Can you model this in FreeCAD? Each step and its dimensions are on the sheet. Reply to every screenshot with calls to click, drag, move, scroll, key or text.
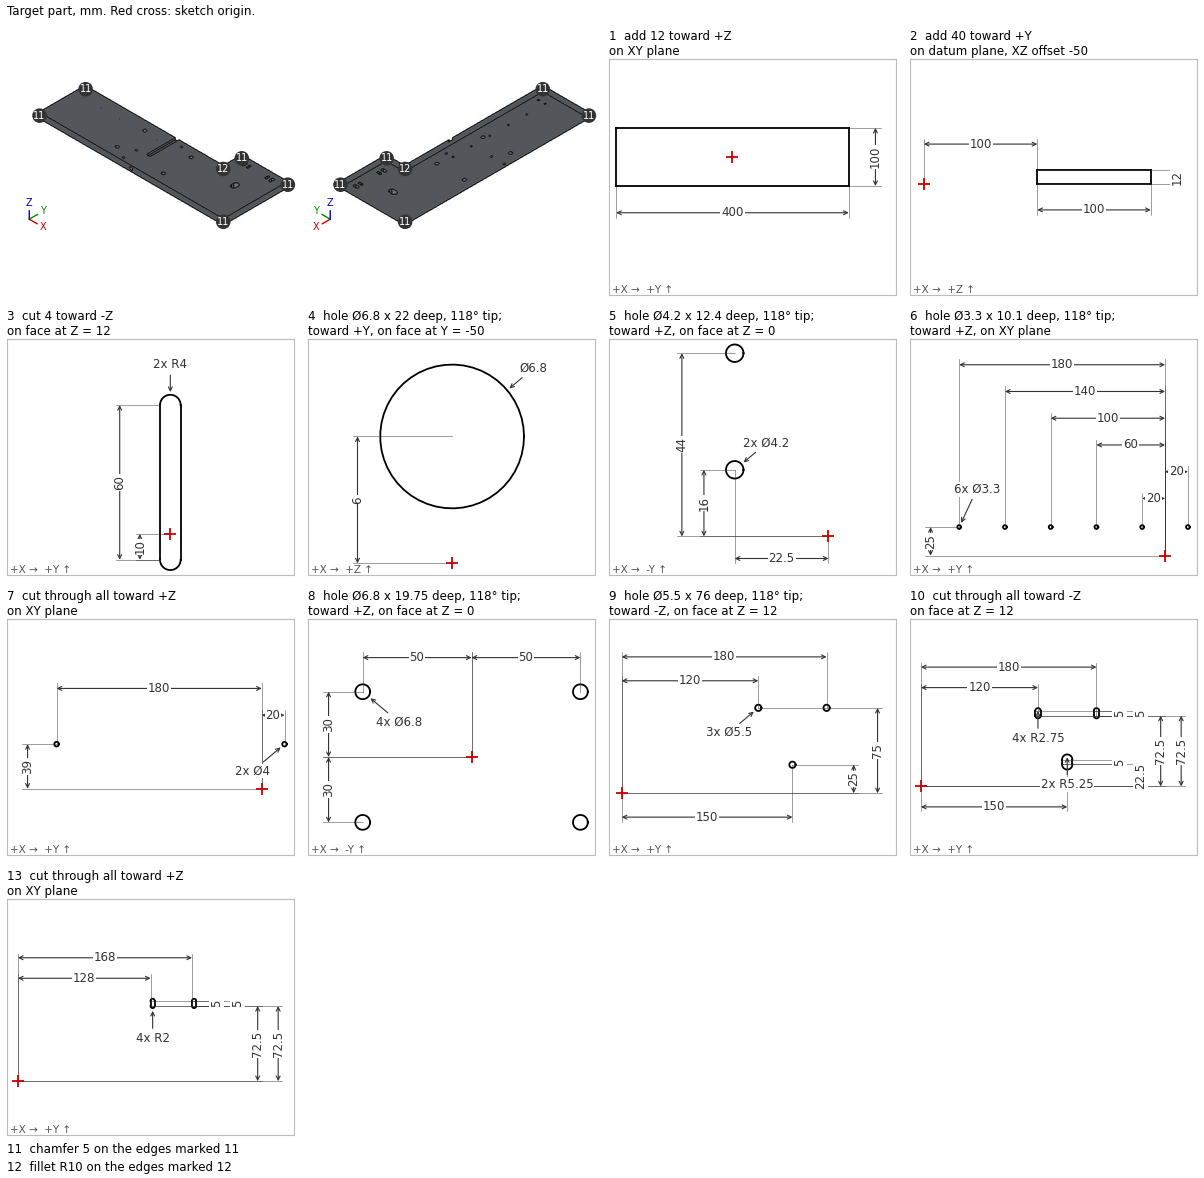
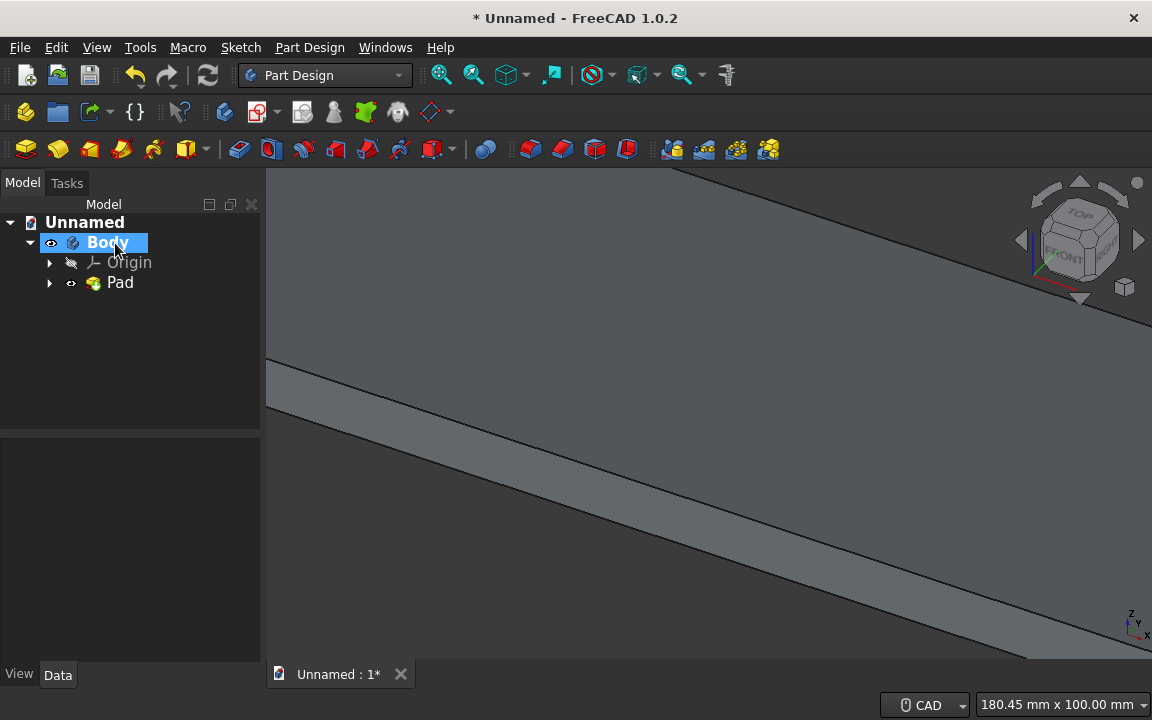
click(442, 76)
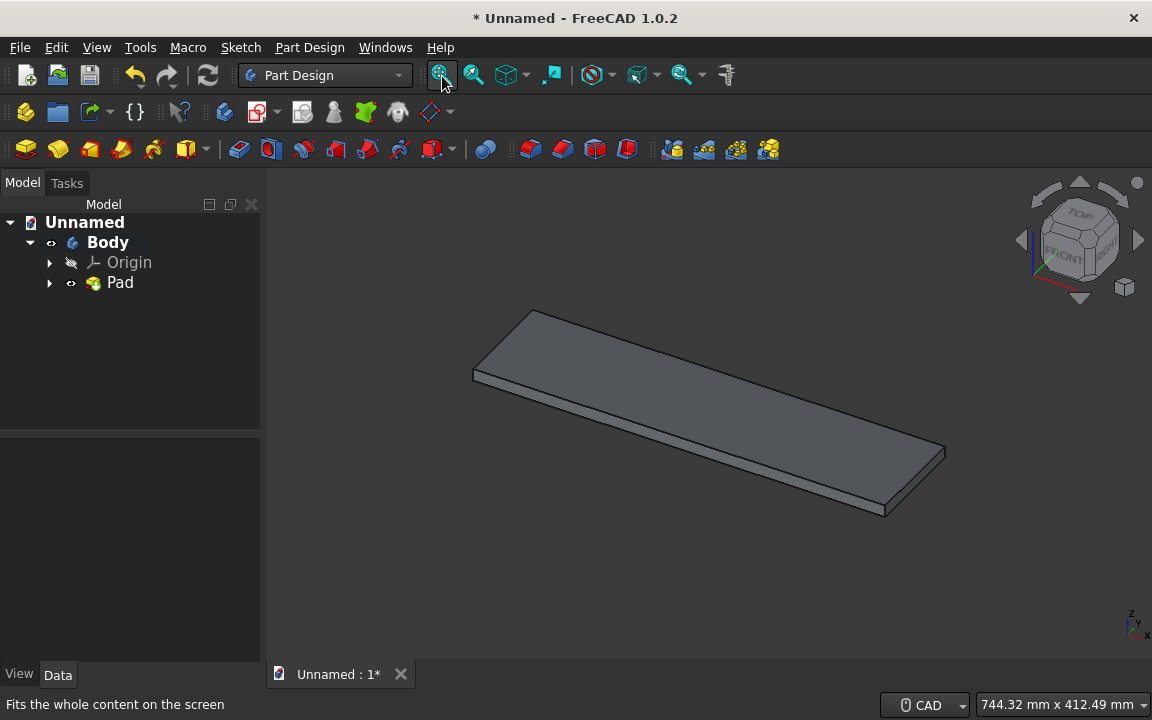
key(4)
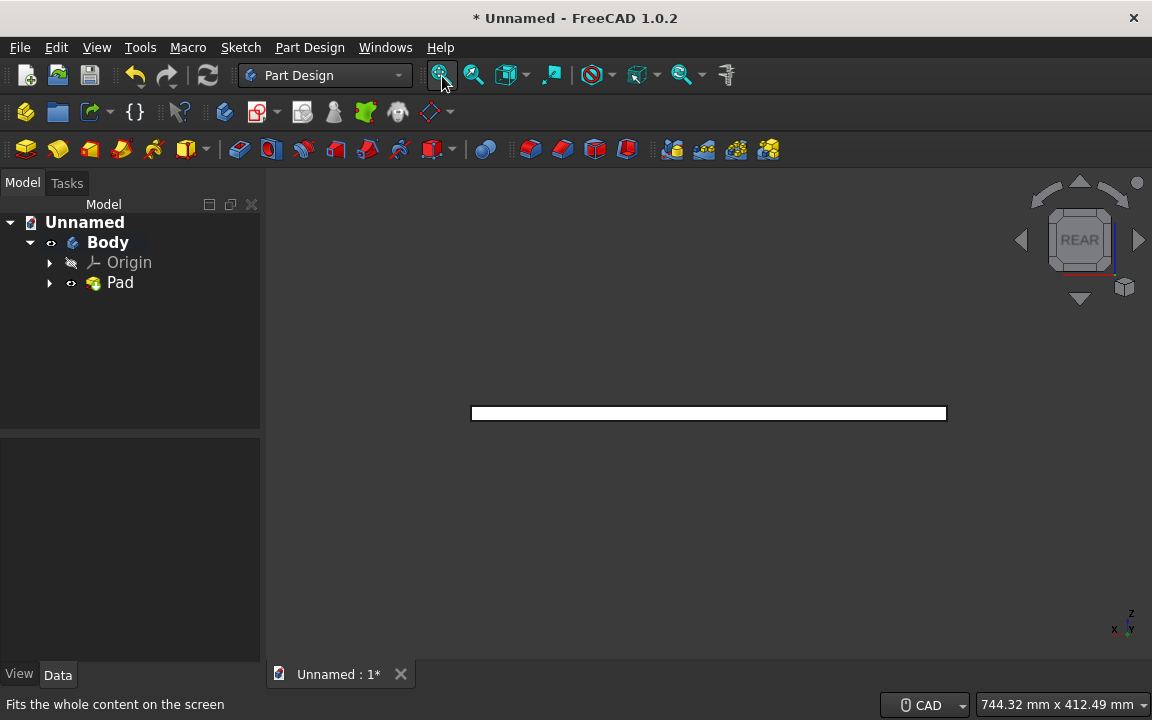
key(2)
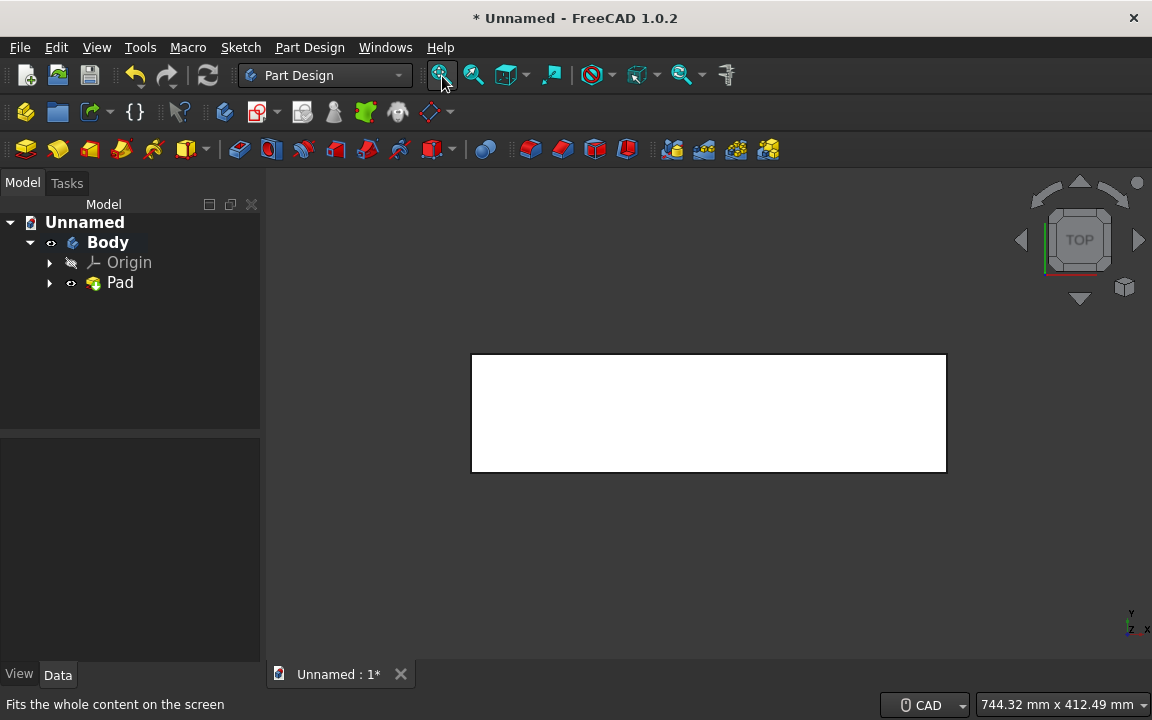
key(3)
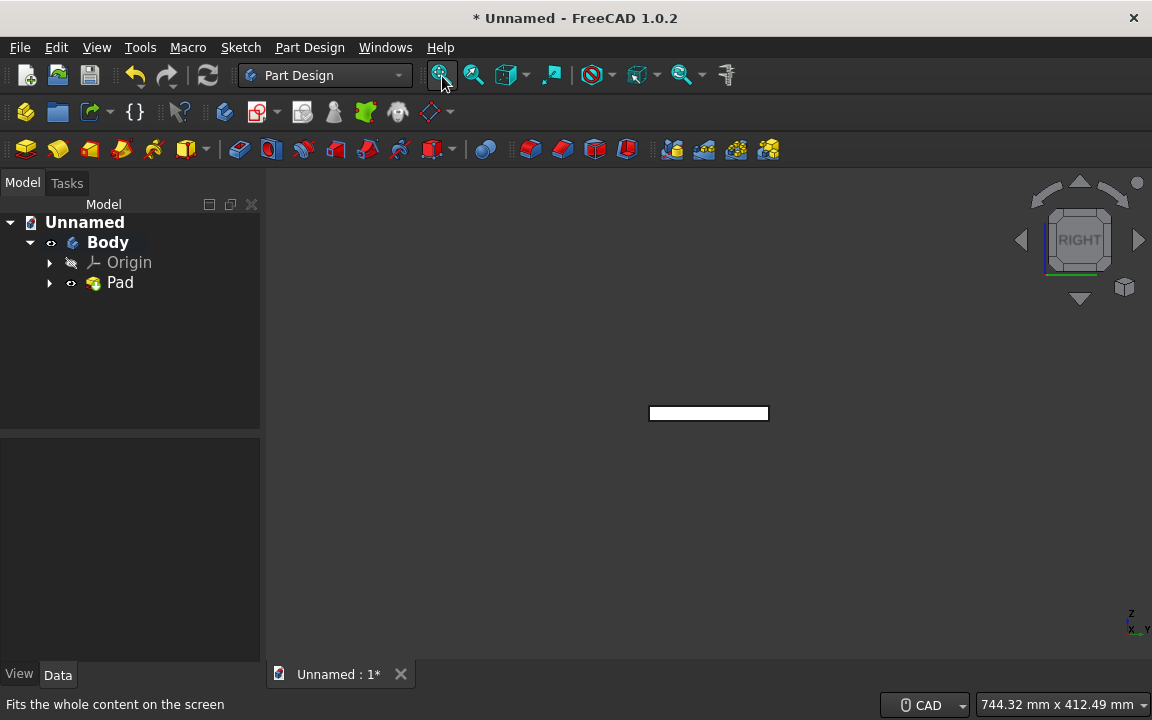
click(442, 76)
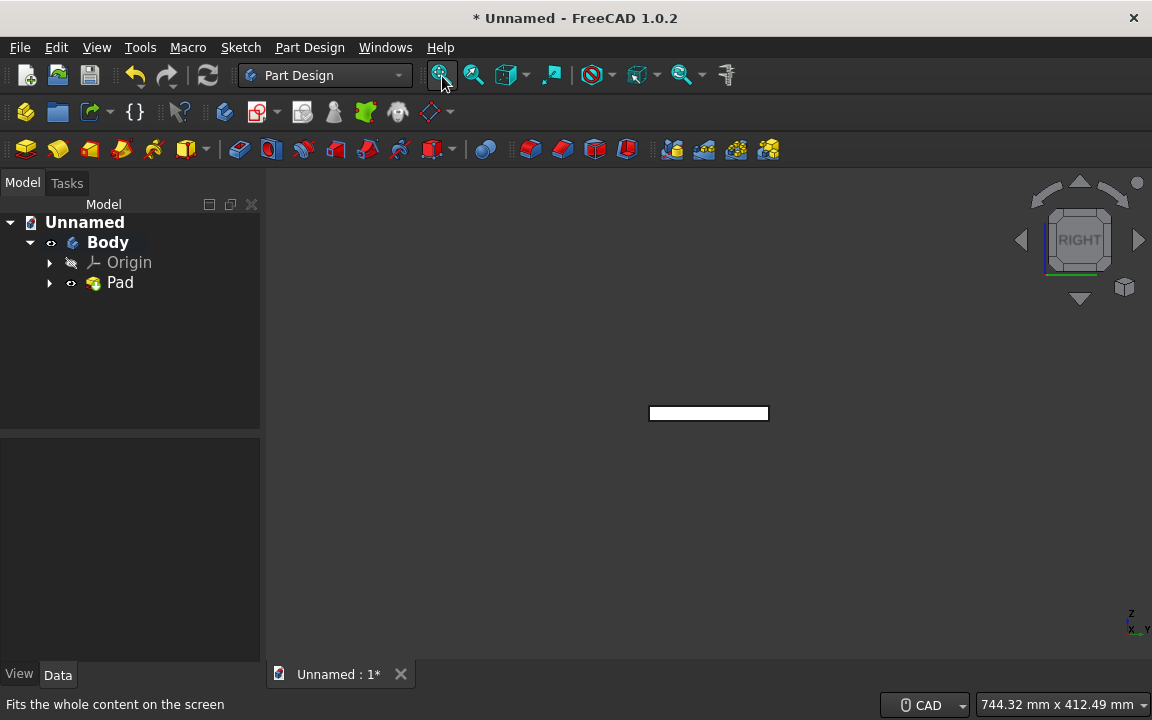
click(50, 263)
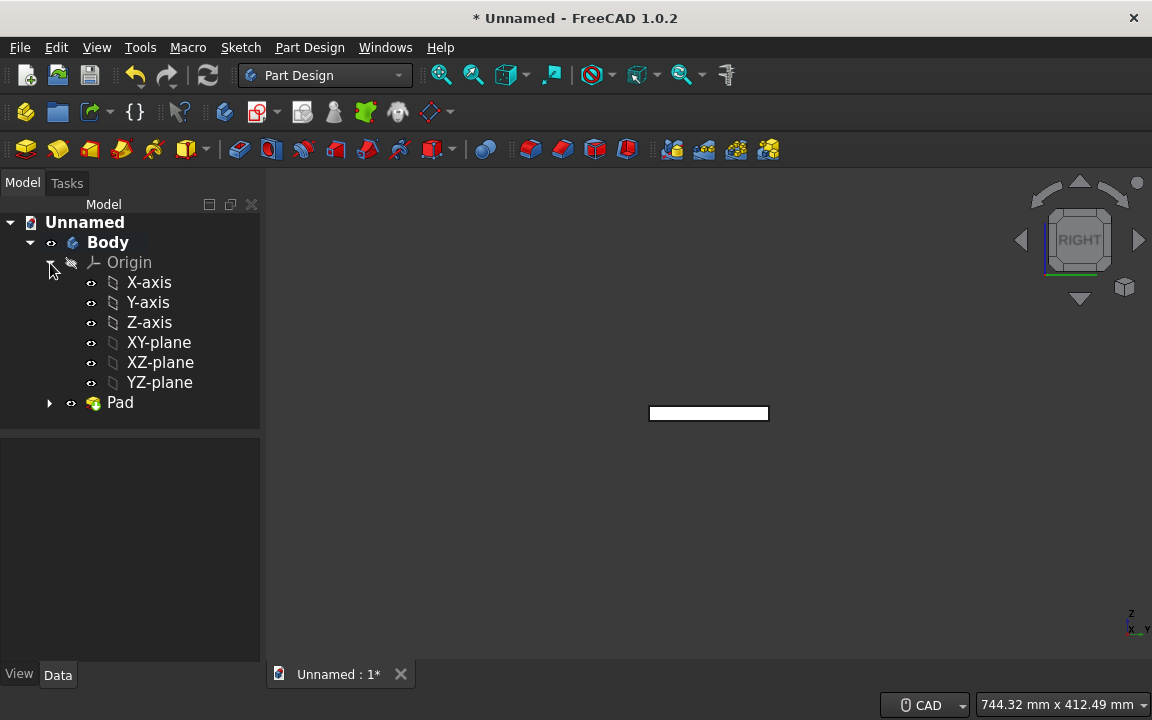
click(136, 363)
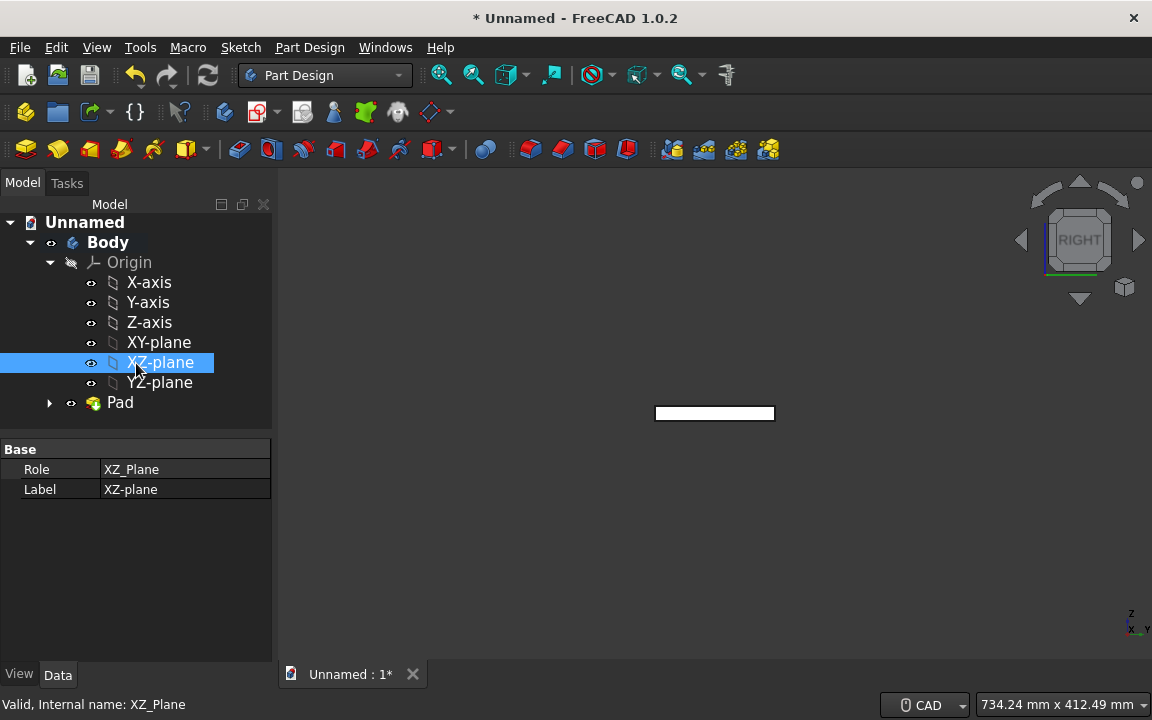
click(430, 112)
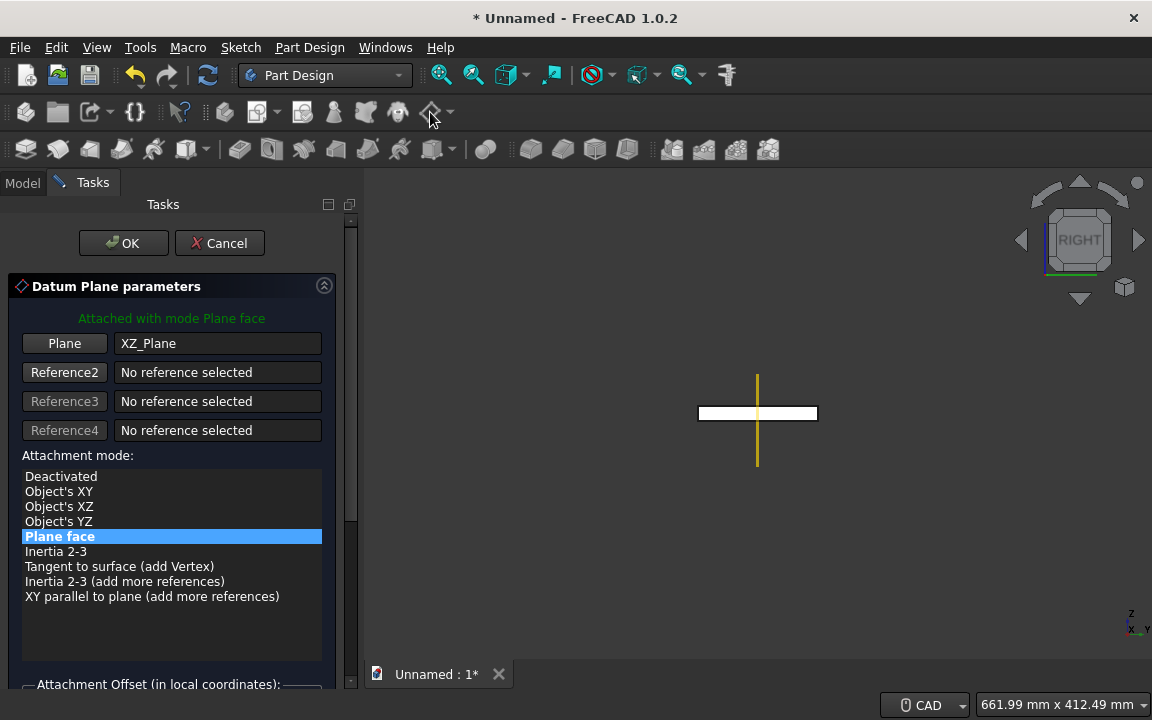
scroll(351, 451, down, 3)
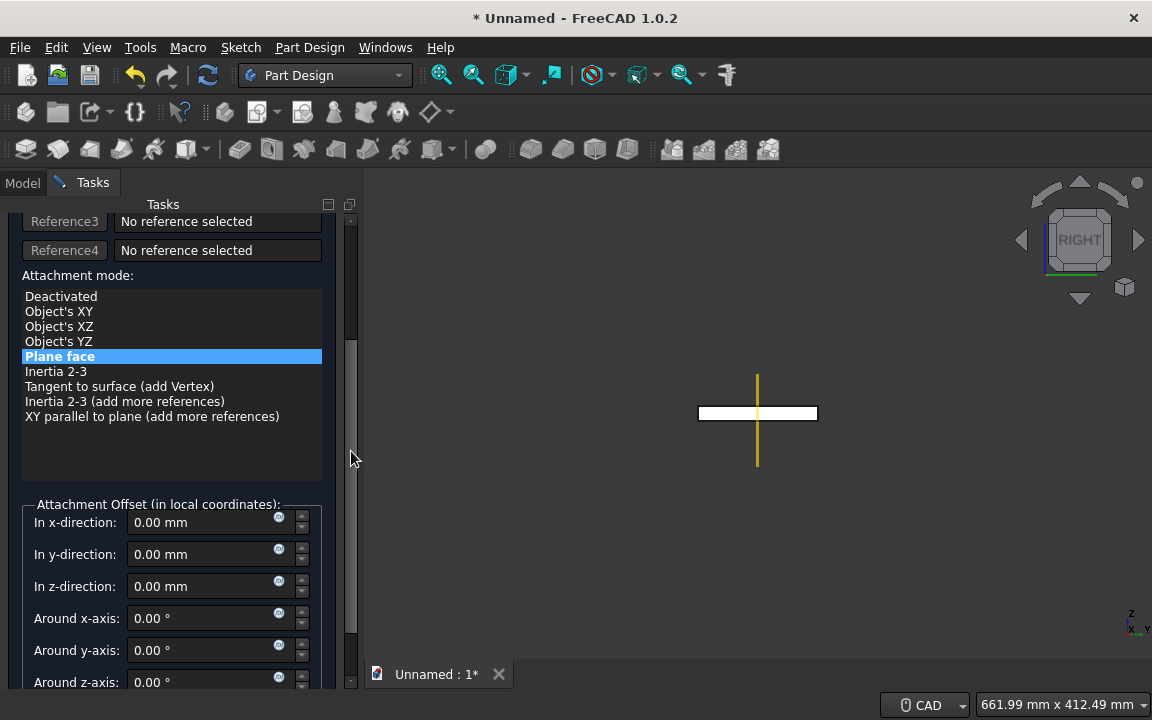
triple_click(210, 586)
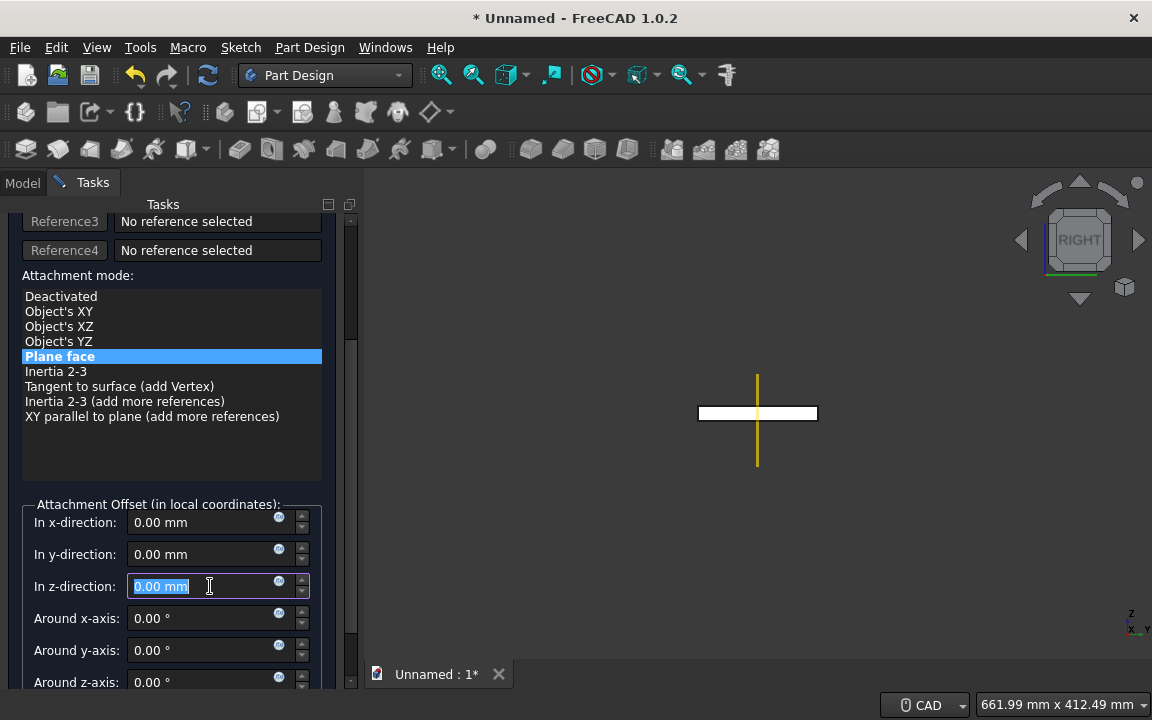
text(-50)
key(Tab)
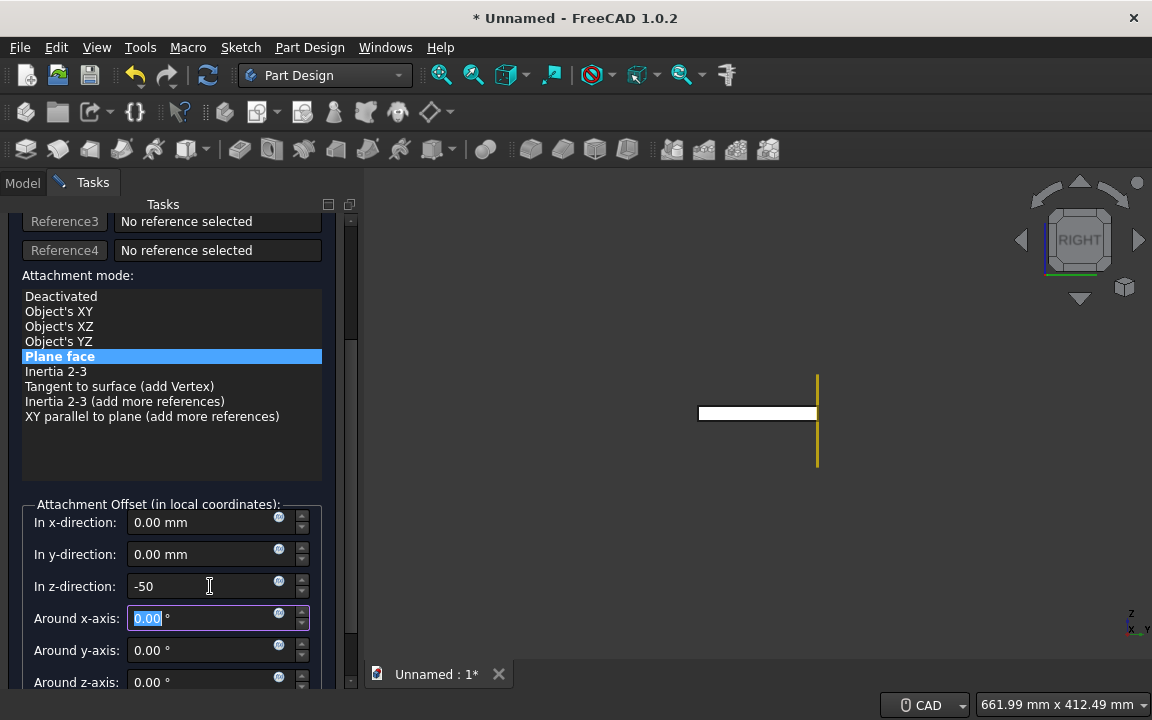
scroll(351, 451, up, 4)